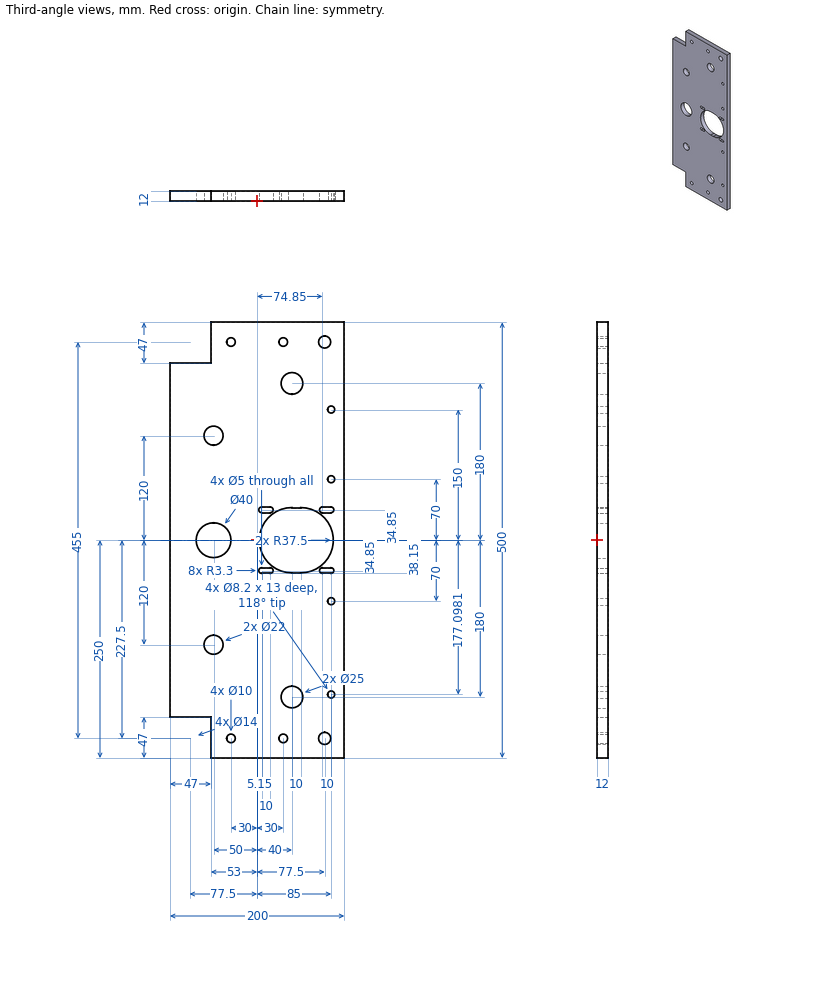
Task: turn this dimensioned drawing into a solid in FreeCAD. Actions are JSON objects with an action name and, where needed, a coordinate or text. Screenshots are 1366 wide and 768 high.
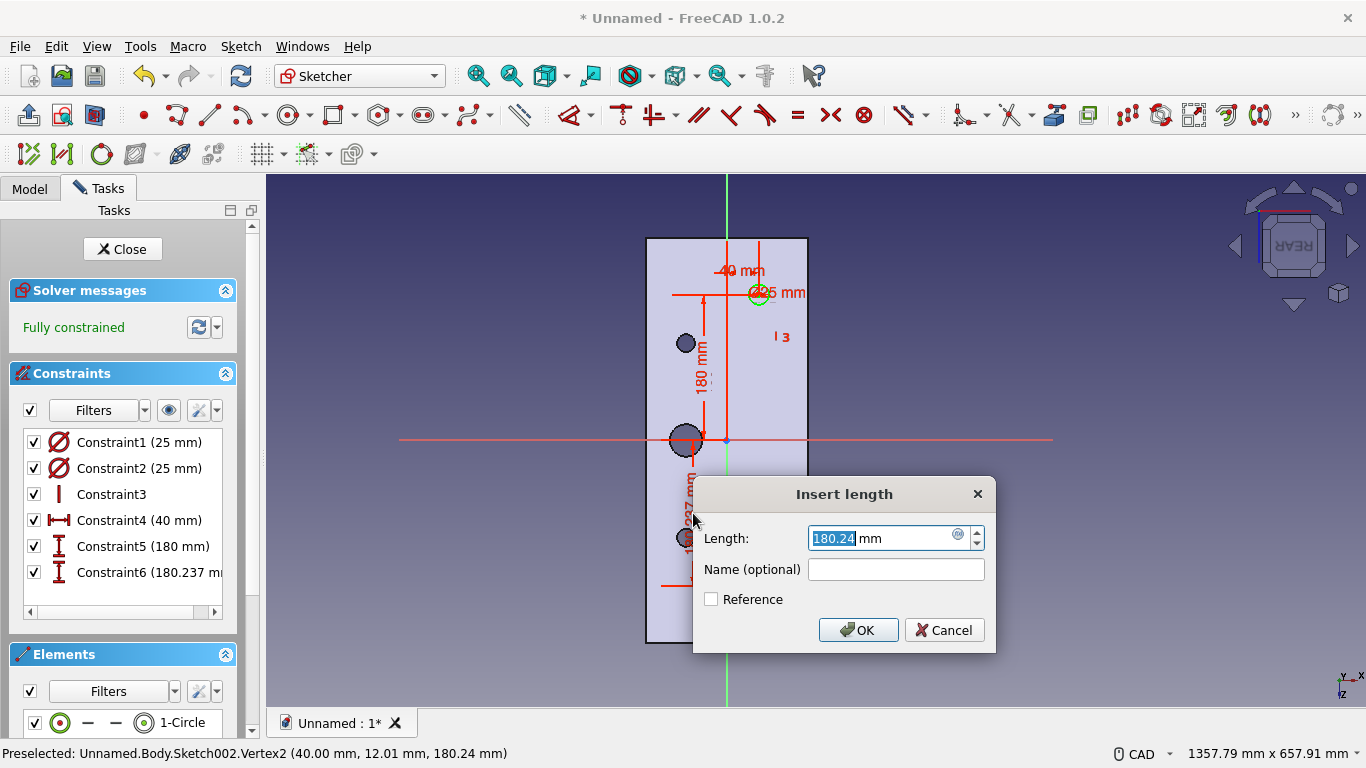
{"action": "type", "text": "180"}
{"action": "key", "text": "Return"}
{"action": "key", "text": "Escape"}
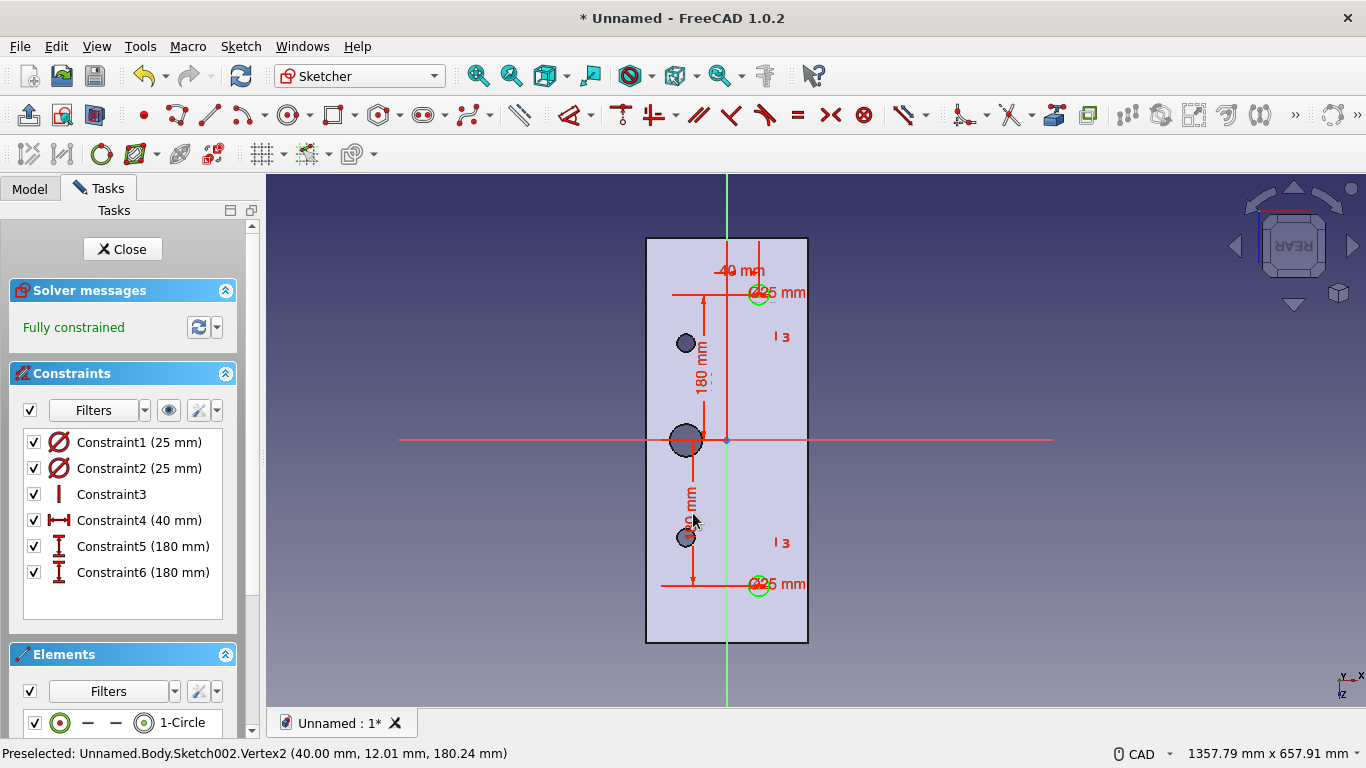
{"action": "left_click", "coordinate": [123, 249]}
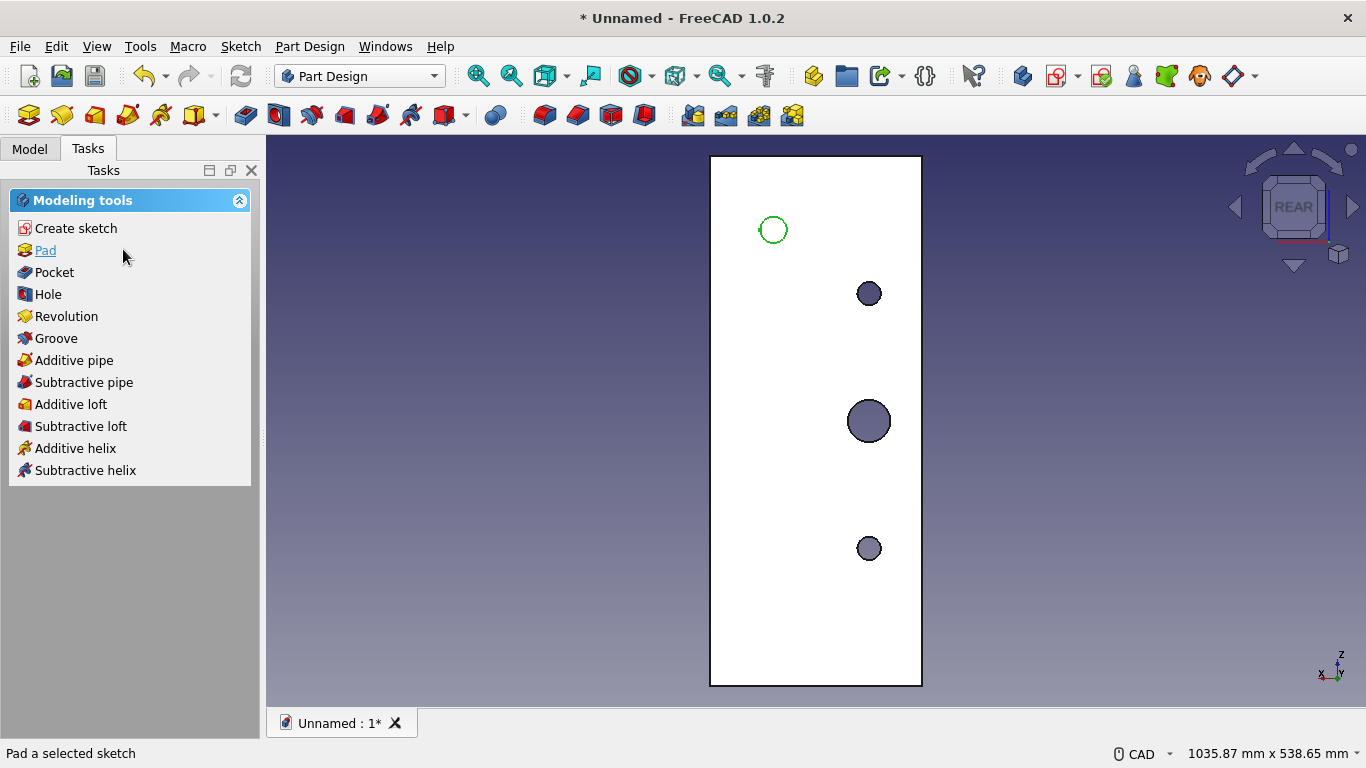
{"action": "left_click", "coordinate": [246, 116]}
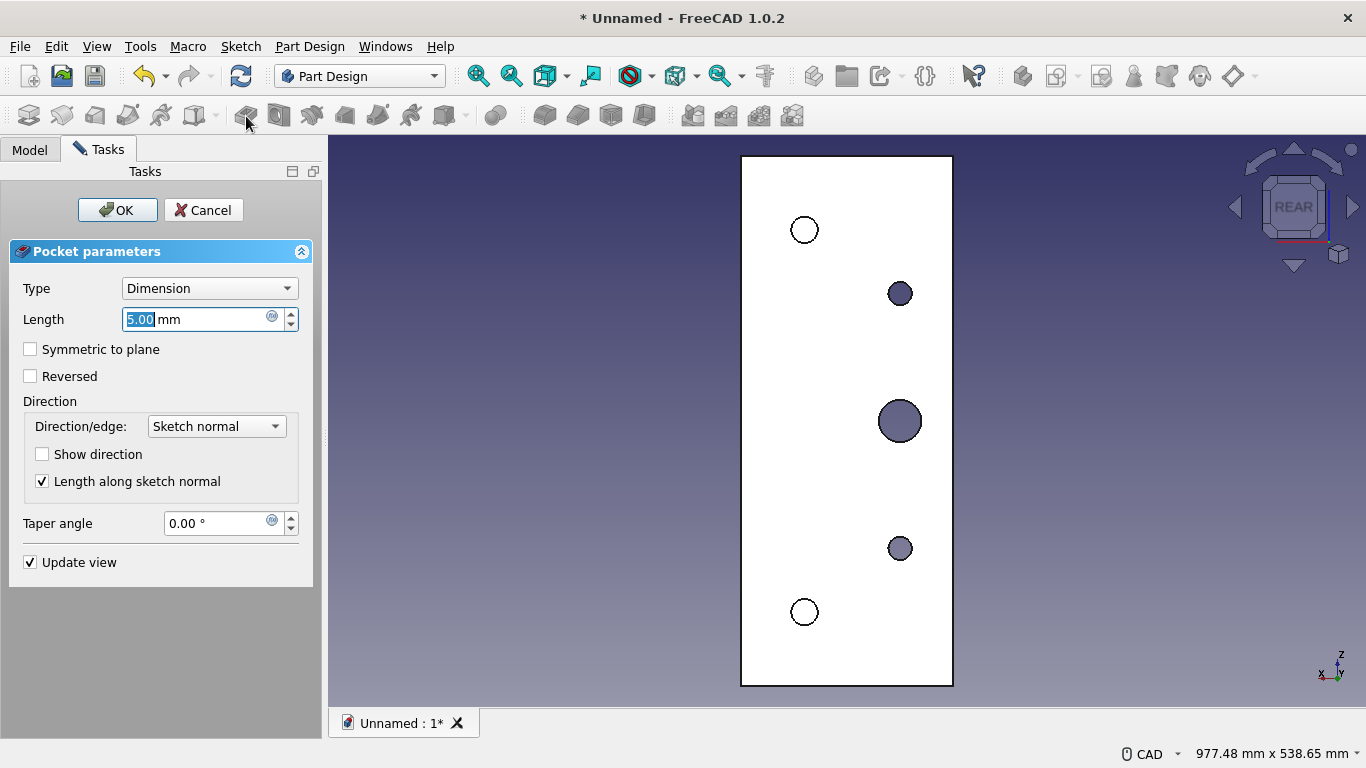
{"action": "type", "text": "12"}
{"action": "key", "text": "Tab"}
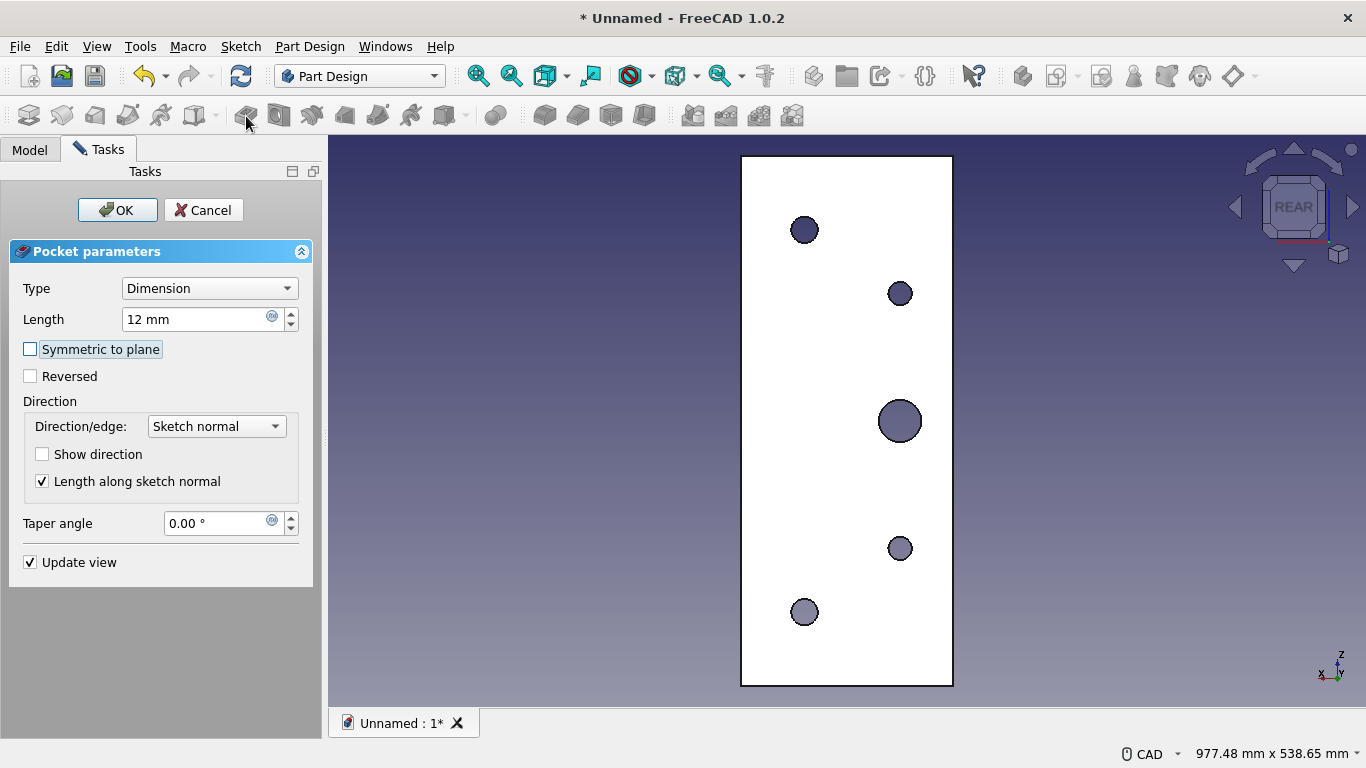
{"action": "left_click", "coordinate": [118, 210]}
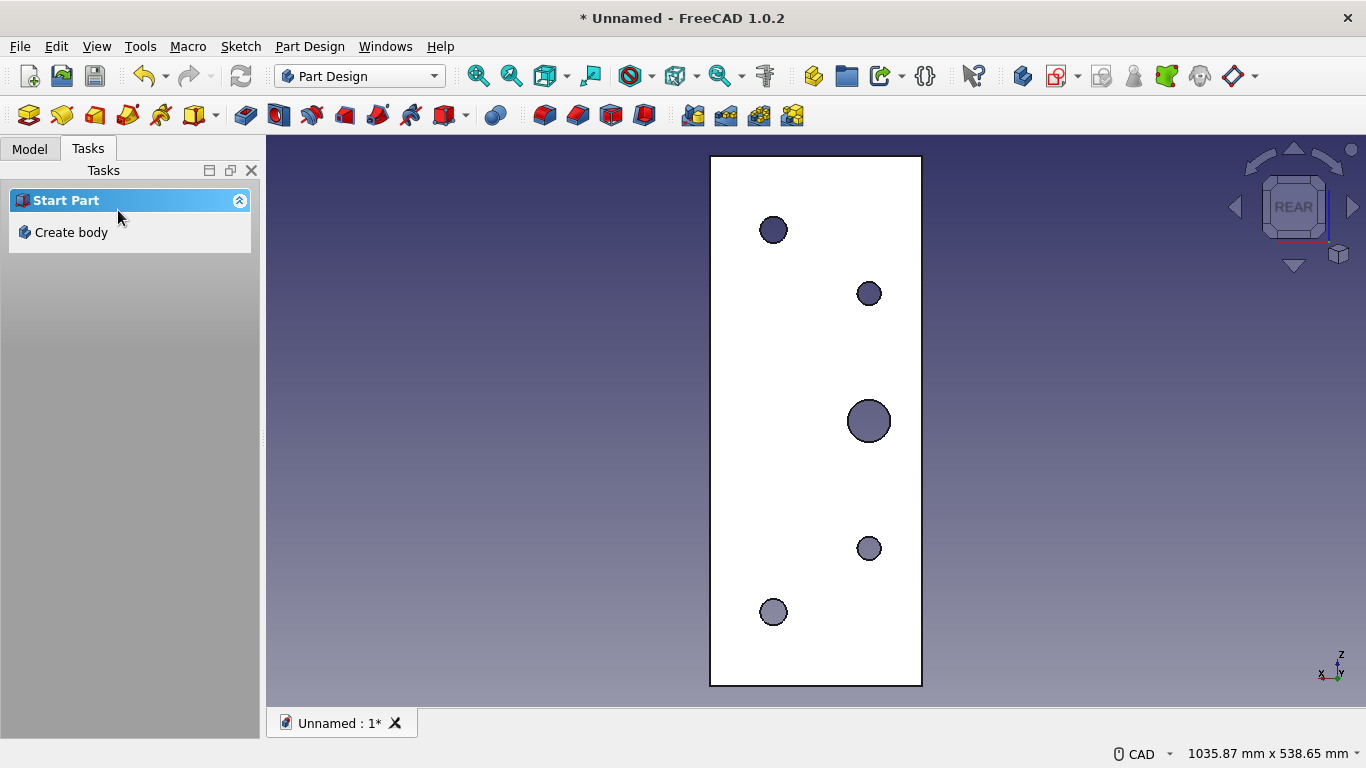
{"action": "left_click", "coordinate": [786, 344]}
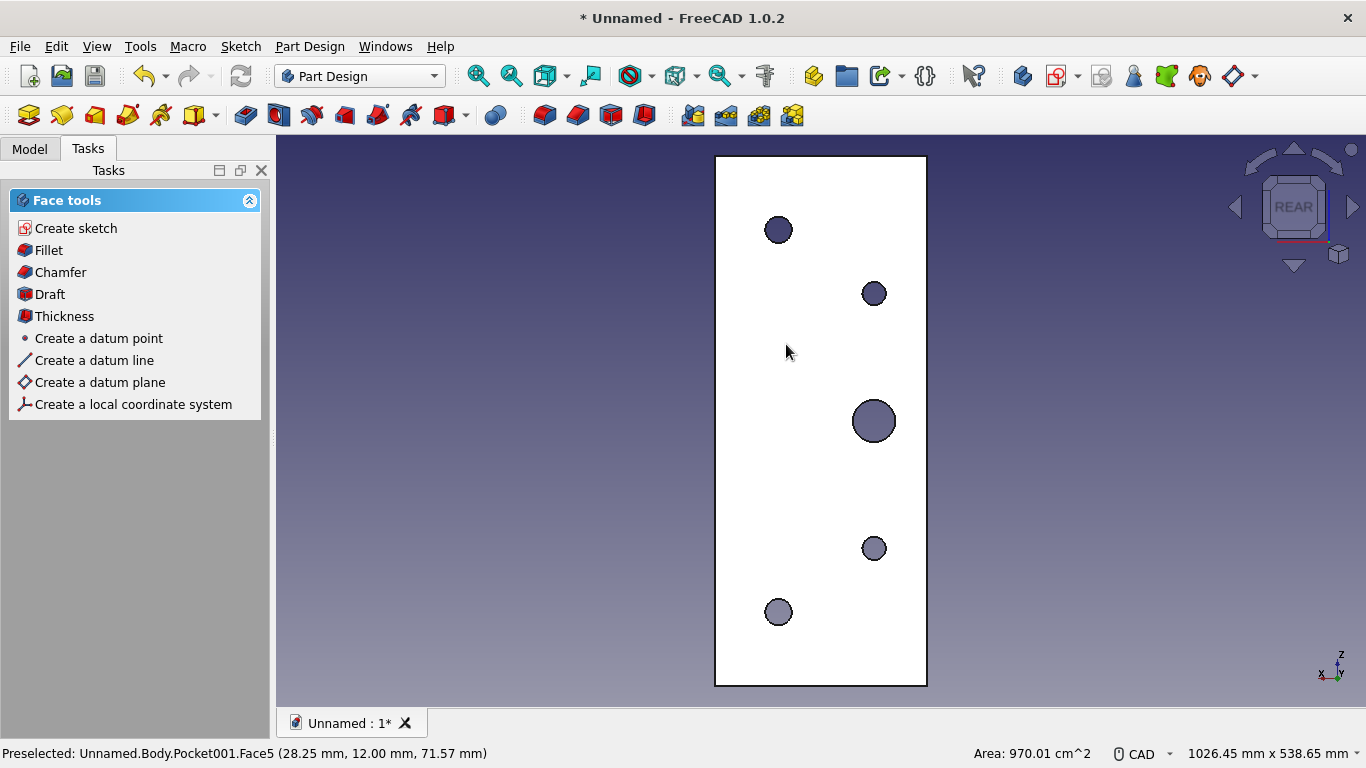
{"action": "left_click", "coordinate": [1056, 76]}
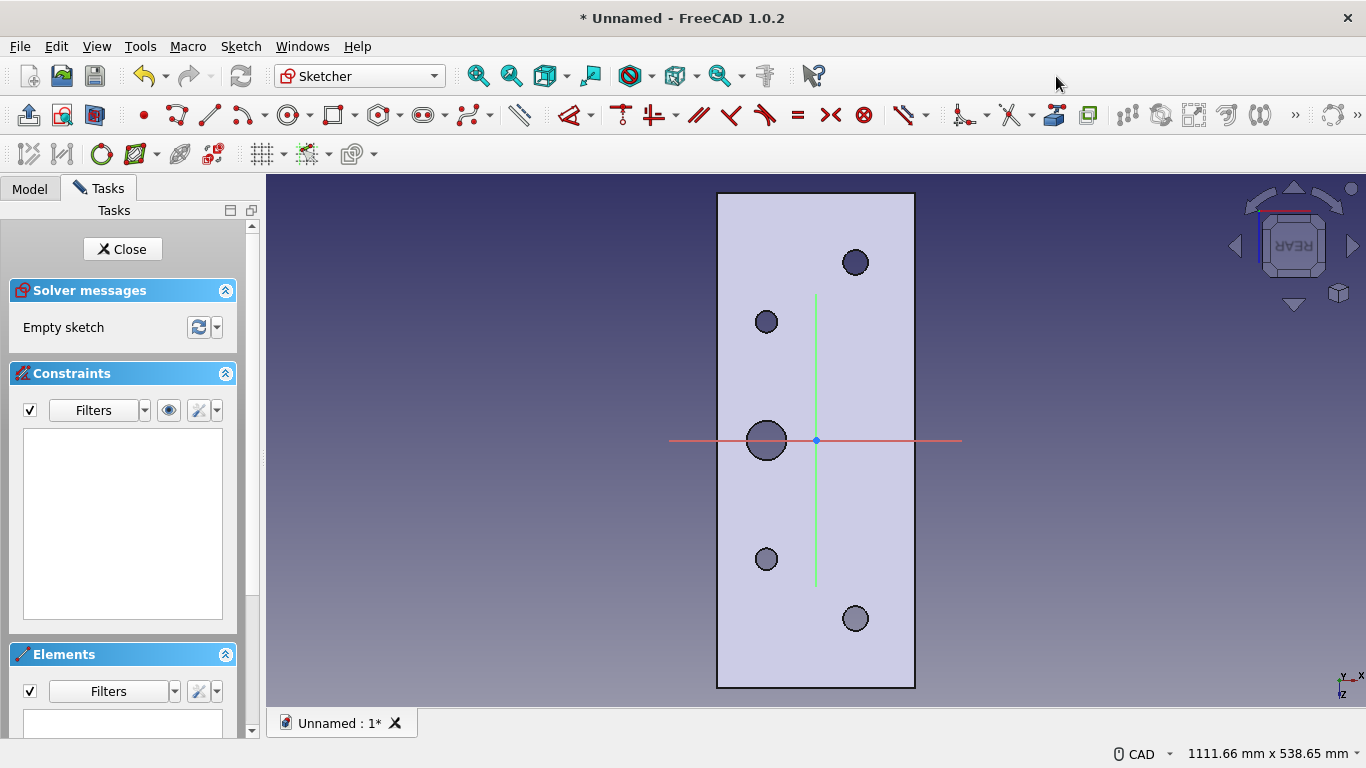
{"action": "scroll", "coordinate": [608, 441], "scroll_direction": "down", "scroll_amount": 2}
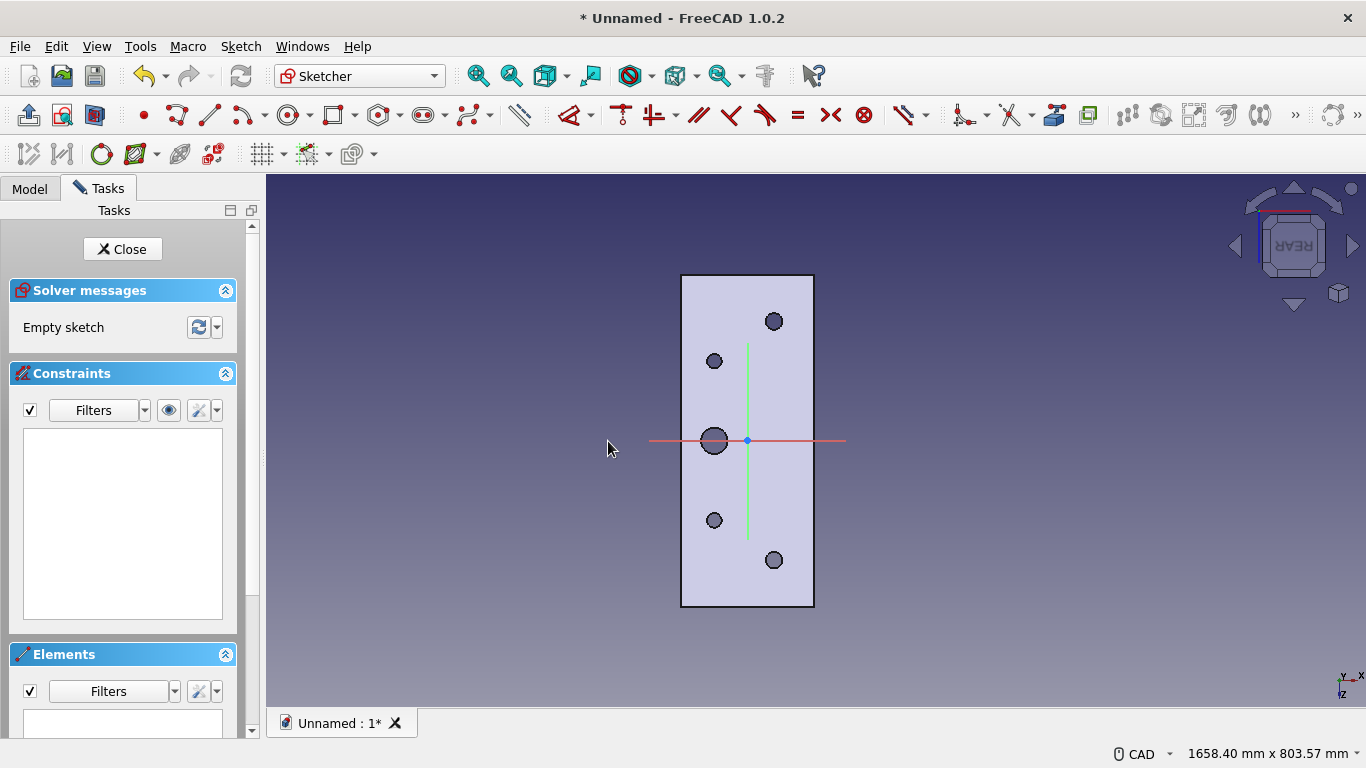
{"action": "left_click", "coordinate": [288, 116]}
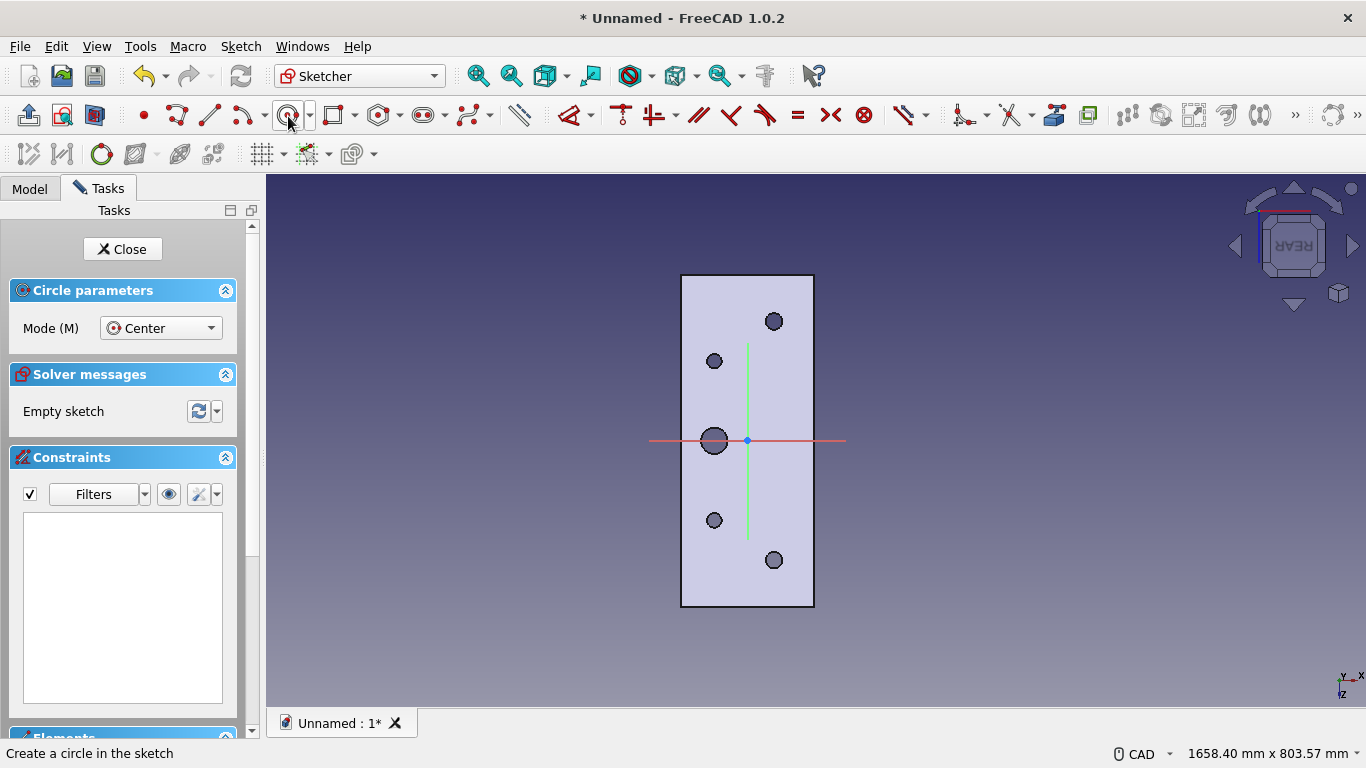
{"action": "scroll", "coordinate": [696, 290], "scroll_direction": "up", "scroll_amount": 8}